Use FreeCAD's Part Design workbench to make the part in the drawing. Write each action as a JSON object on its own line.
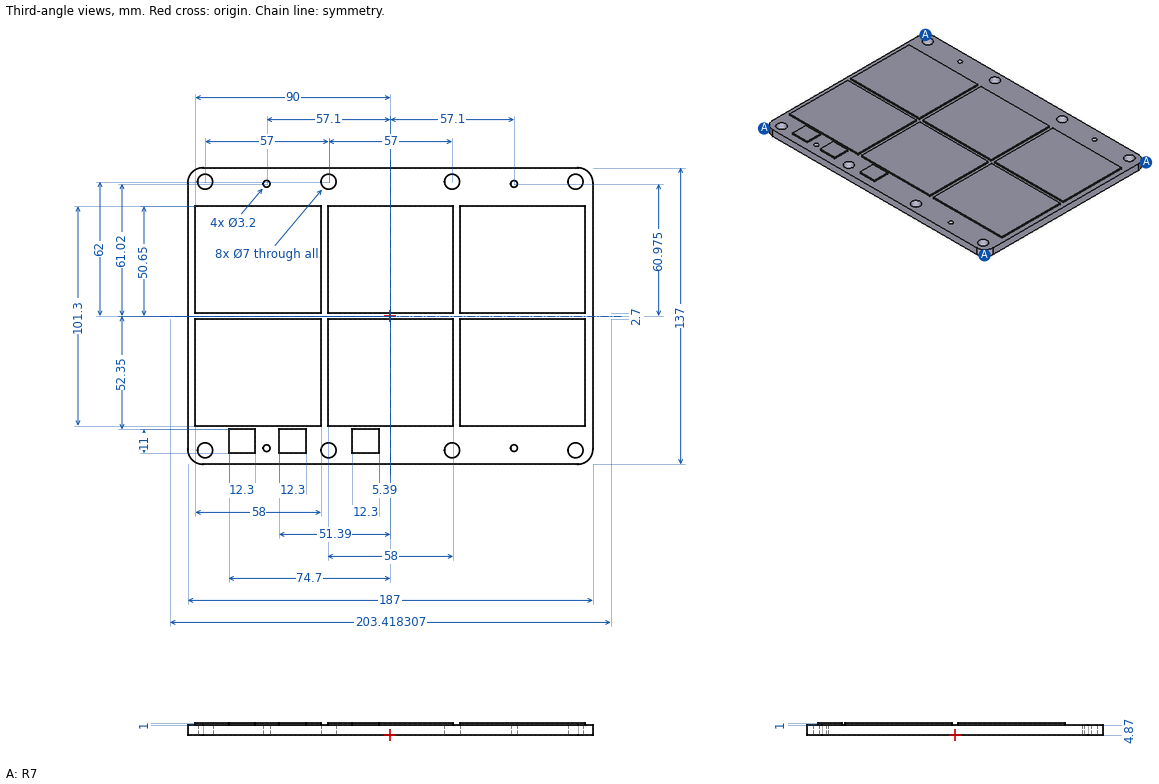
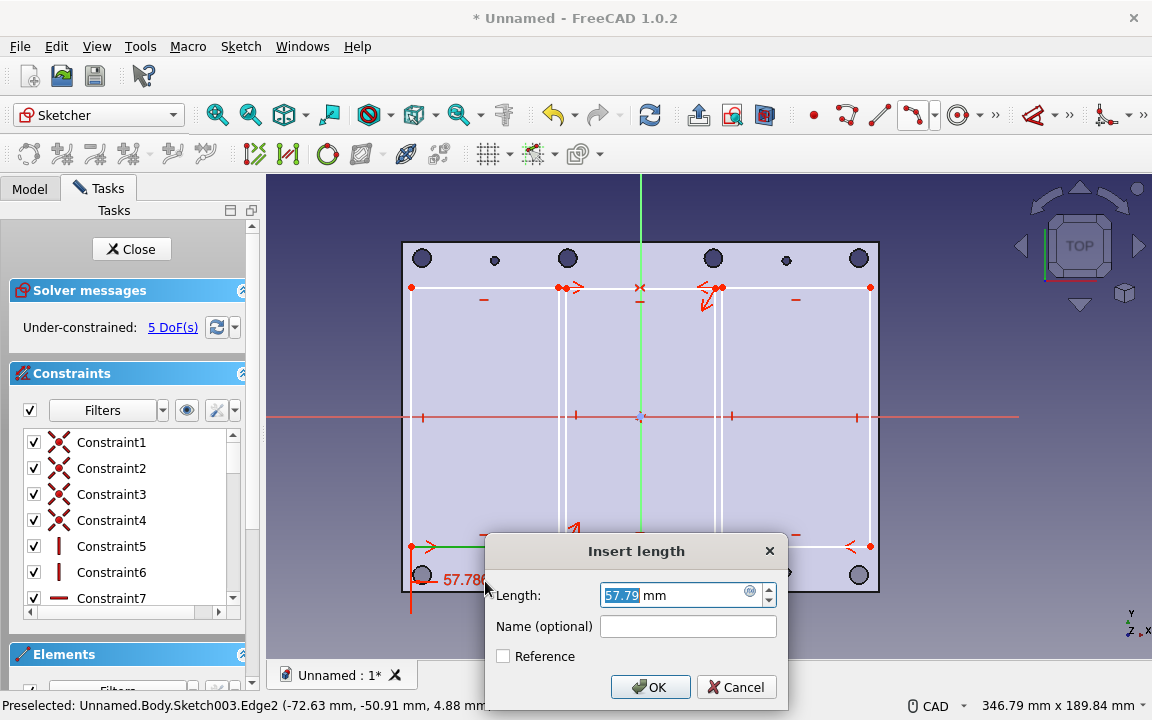
{"action": "type", "text": "58"}
{"action": "key", "text": "Return"}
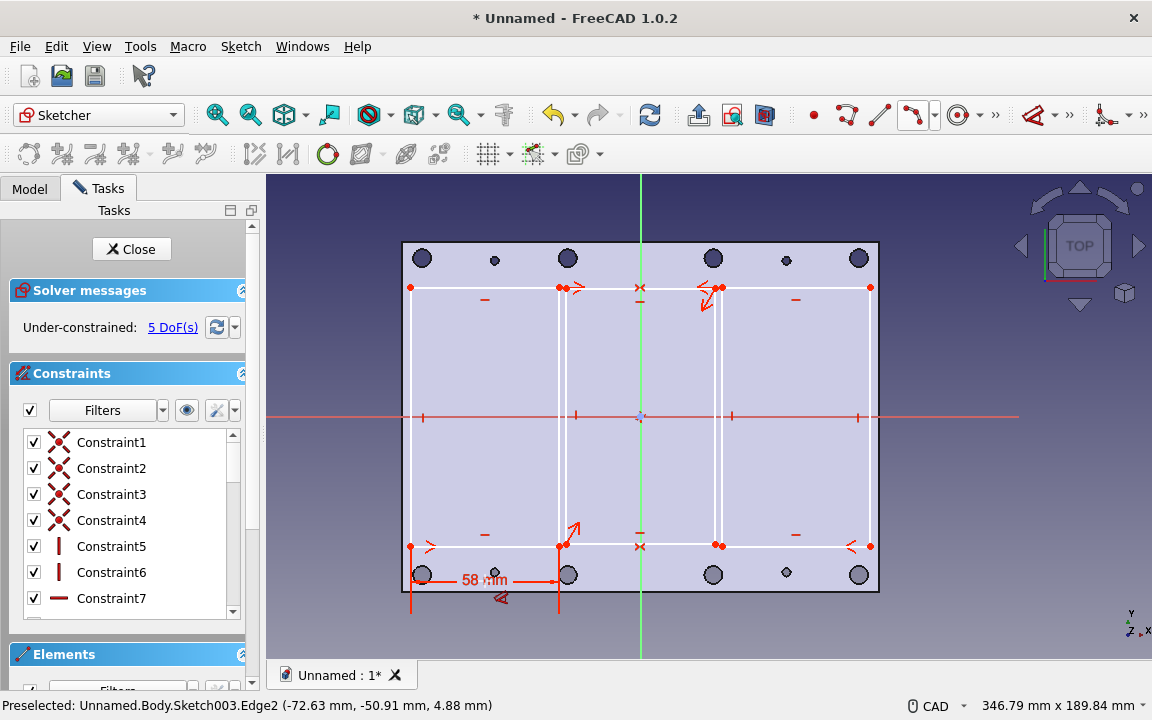
{"action": "left_click", "coordinate": [611, 544]}
{"action": "left_click", "coordinate": [606, 578]}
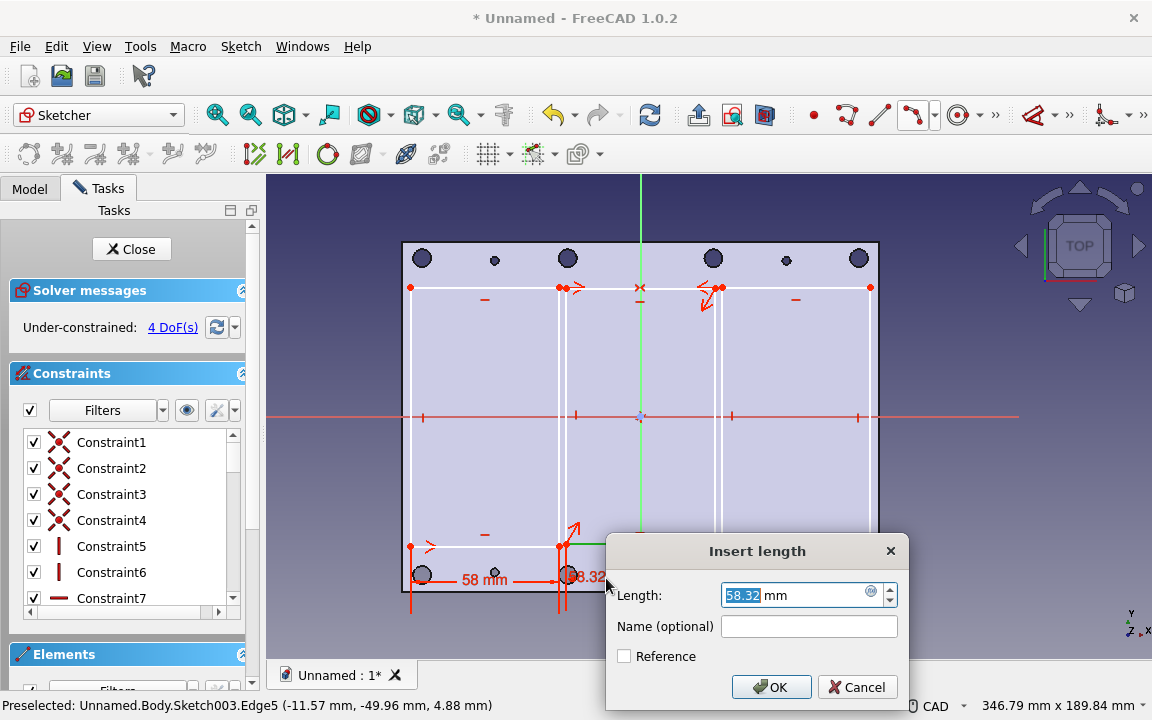
{"action": "type", "text": "58"}
{"action": "key", "text": "Return"}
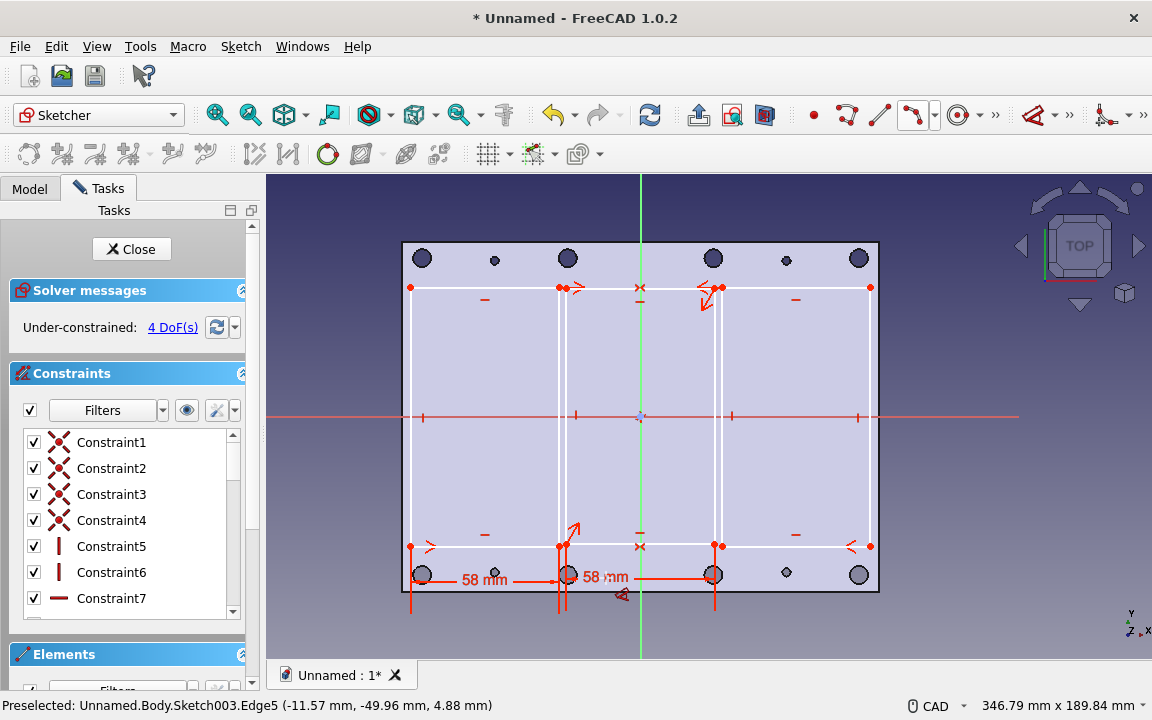
{"action": "left_click", "coordinate": [411, 288]}
{"action": "left_click", "coordinate": [526, 254]}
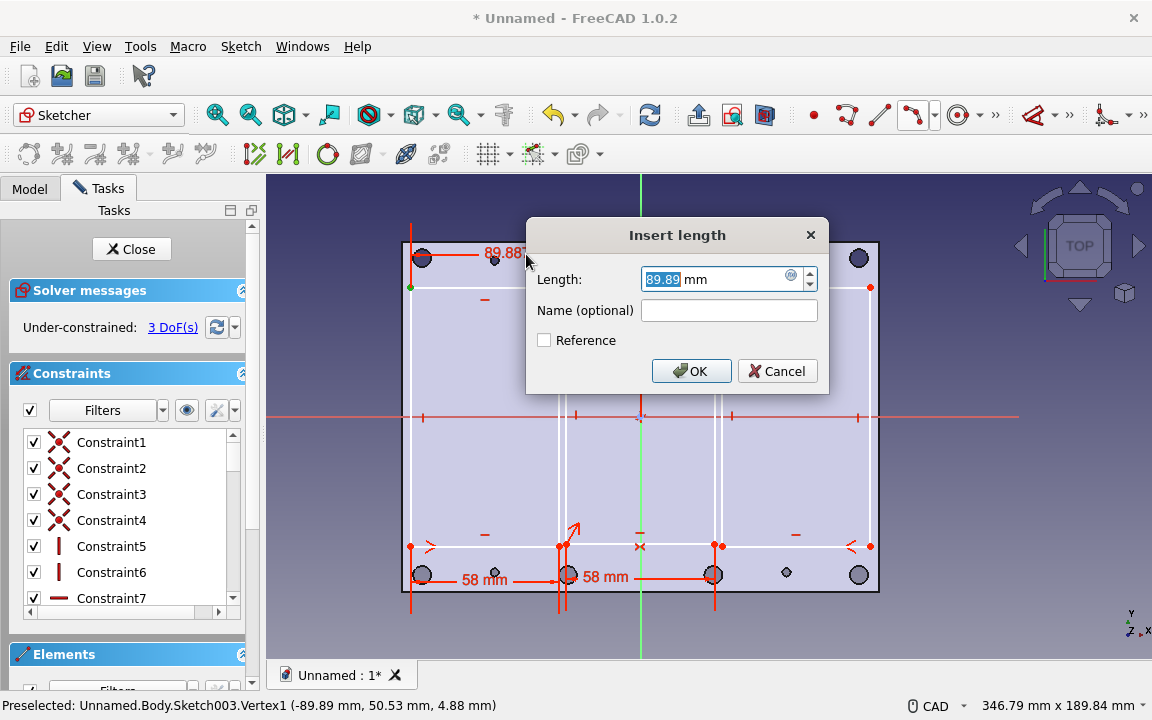
{"action": "type", "text": "90"}
{"action": "key", "text": "Return"}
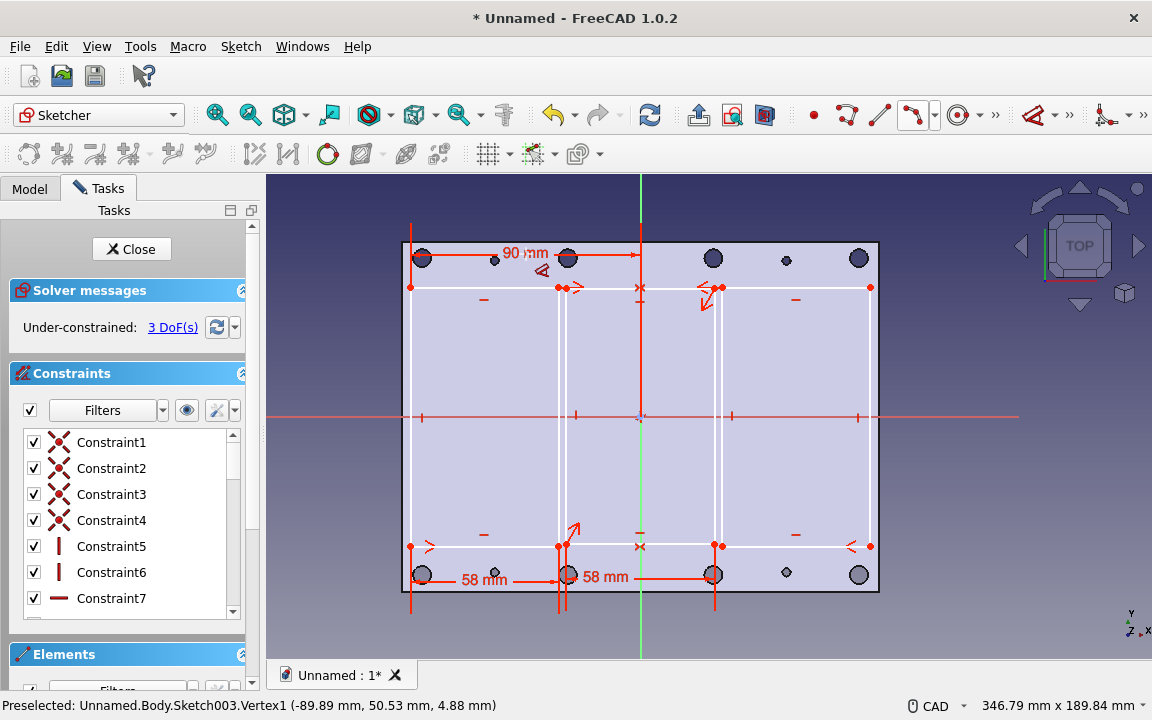
{"action": "left_click", "coordinate": [411, 365]}
{"action": "left_click", "coordinate": [377, 358]}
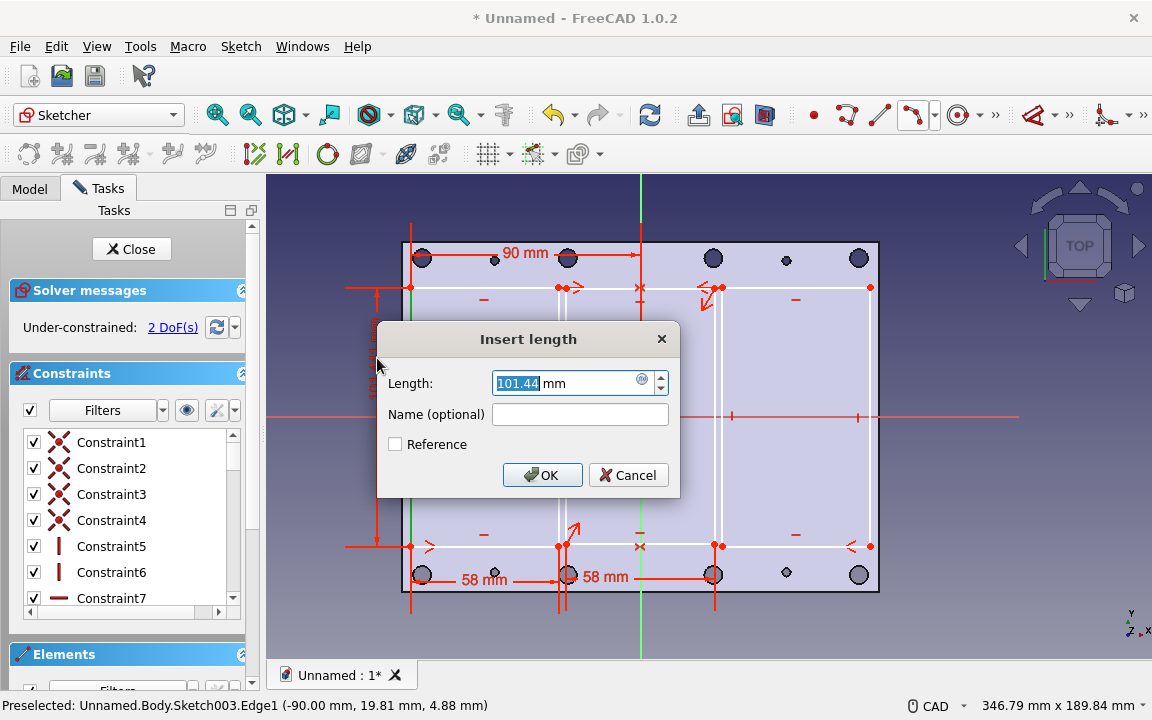
{"action": "type", "text": "101.3"}
{"action": "key", "text": "Return"}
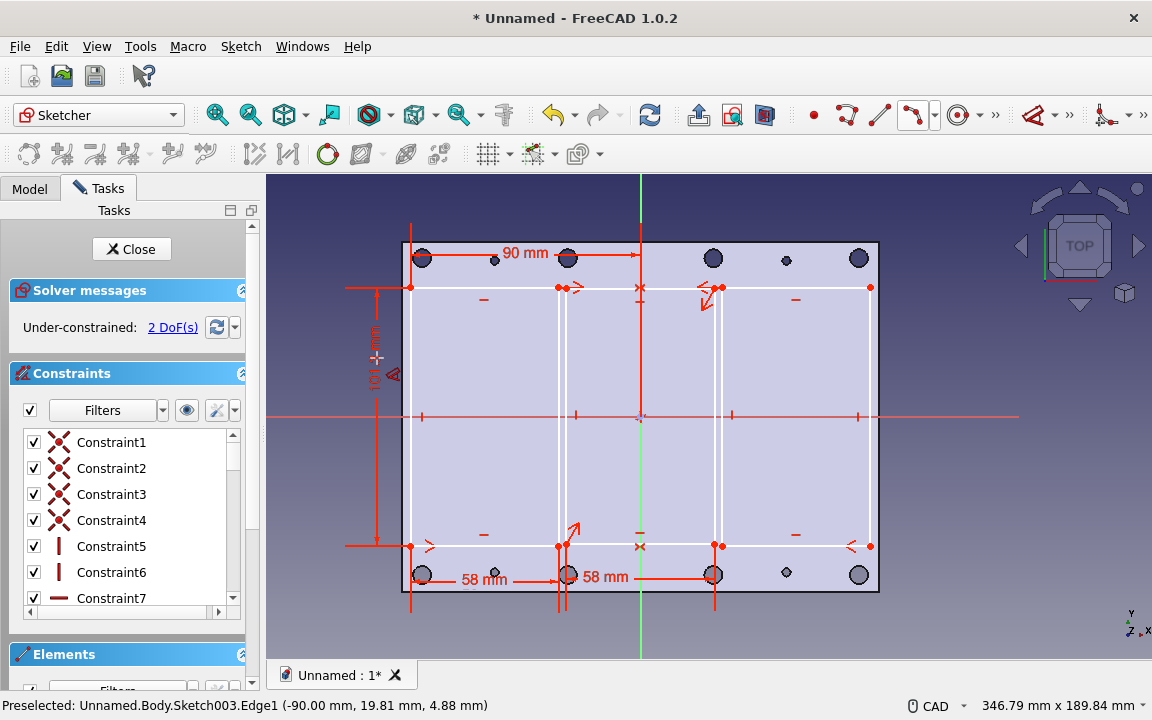
{"action": "scroll", "coordinate": [715, 468], "scroll_direction": "up", "scroll_amount": 3}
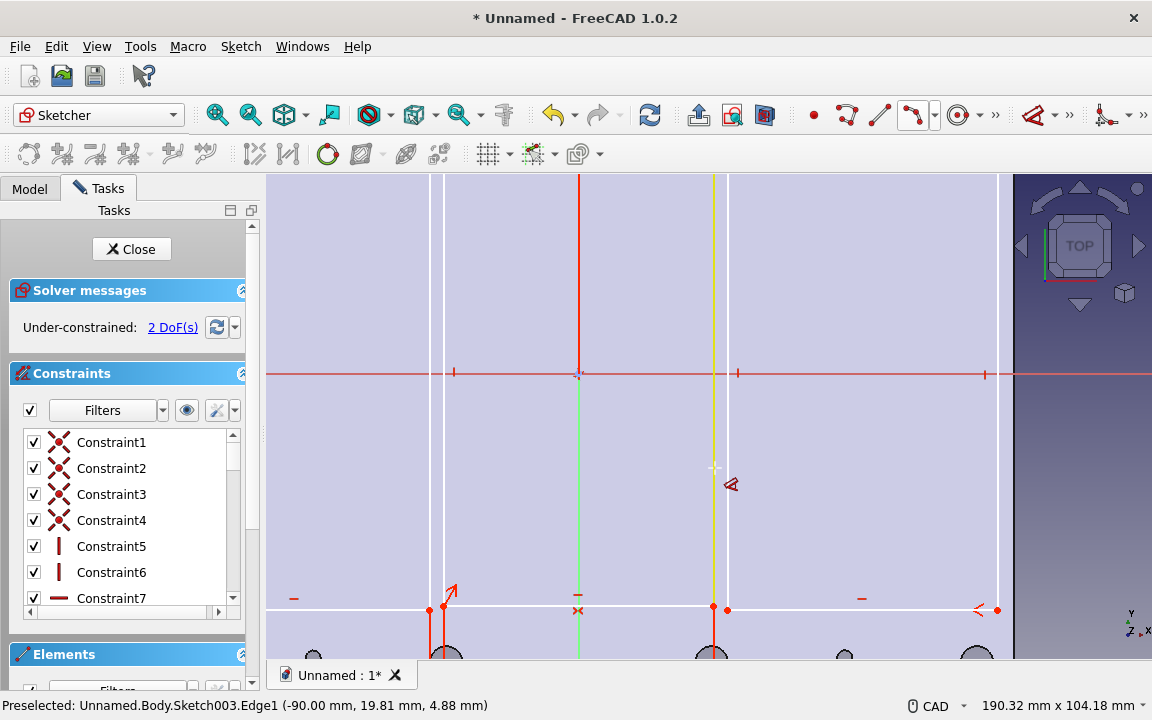
{"action": "left_click", "coordinate": [714, 467]}
{"action": "left_click", "coordinate": [748, 404]}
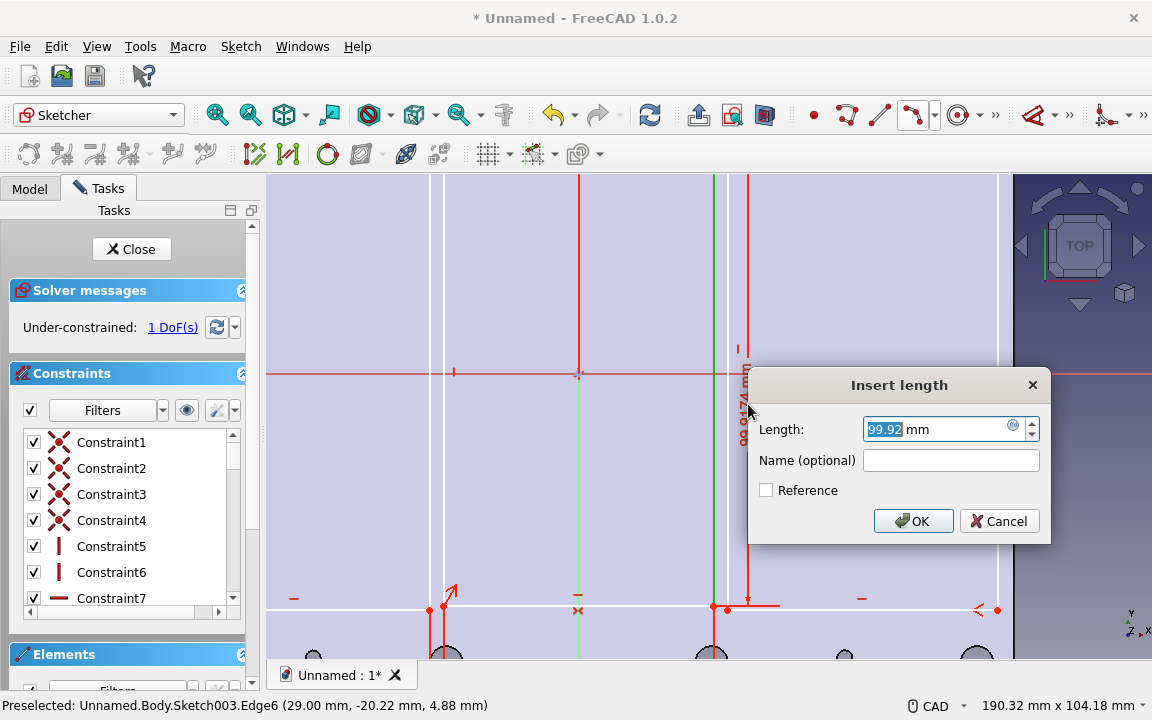
{"action": "type", "text": "101.3"}
{"action": "key", "text": "Return"}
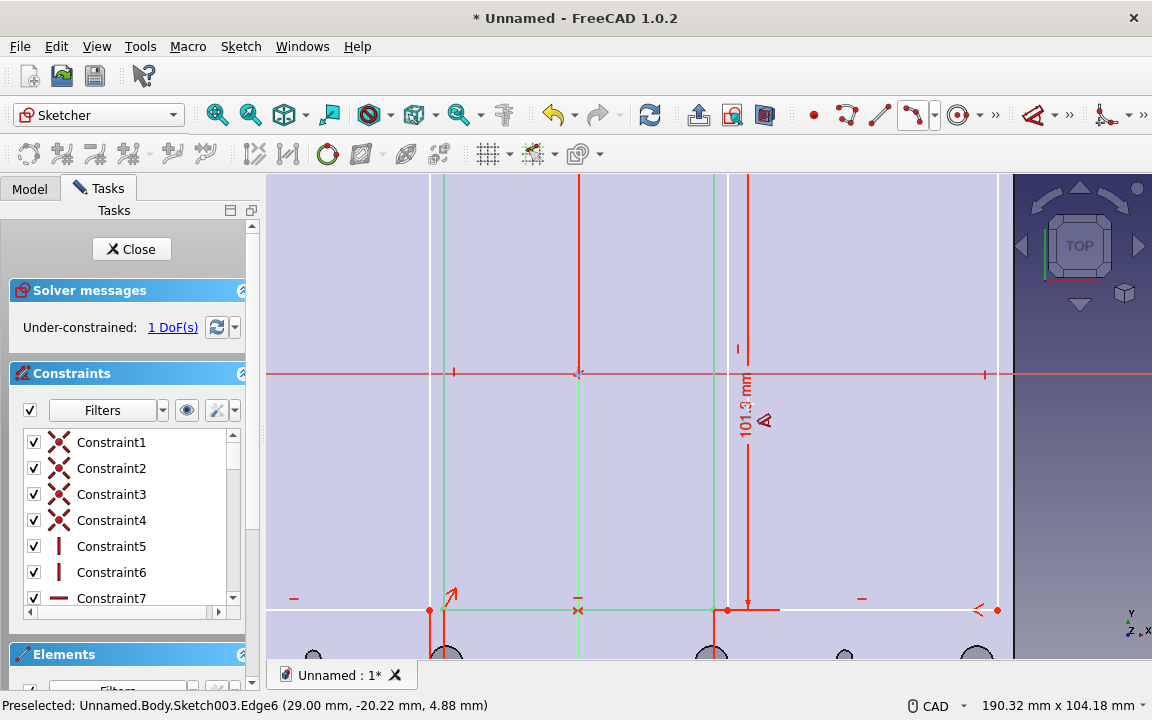
{"action": "scroll", "coordinate": [715, 468], "scroll_direction": "down", "scroll_amount": 3}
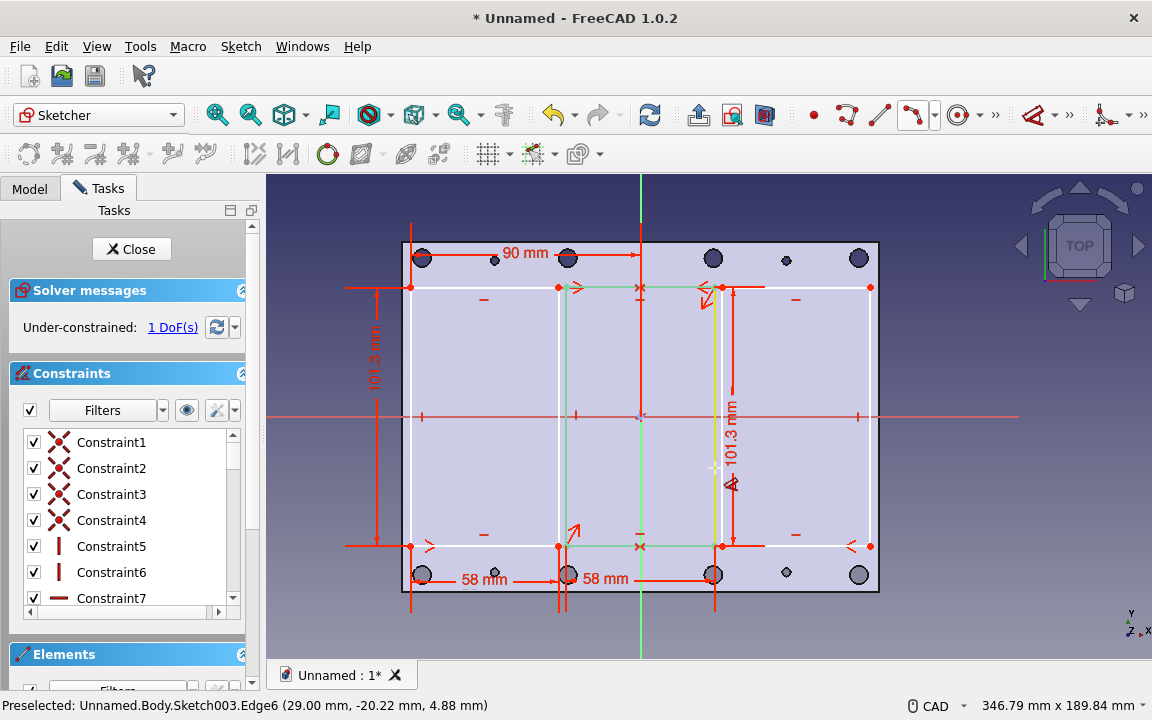
{"action": "left_click", "coordinate": [411, 288]}
{"action": "left_click", "coordinate": [377, 322]}